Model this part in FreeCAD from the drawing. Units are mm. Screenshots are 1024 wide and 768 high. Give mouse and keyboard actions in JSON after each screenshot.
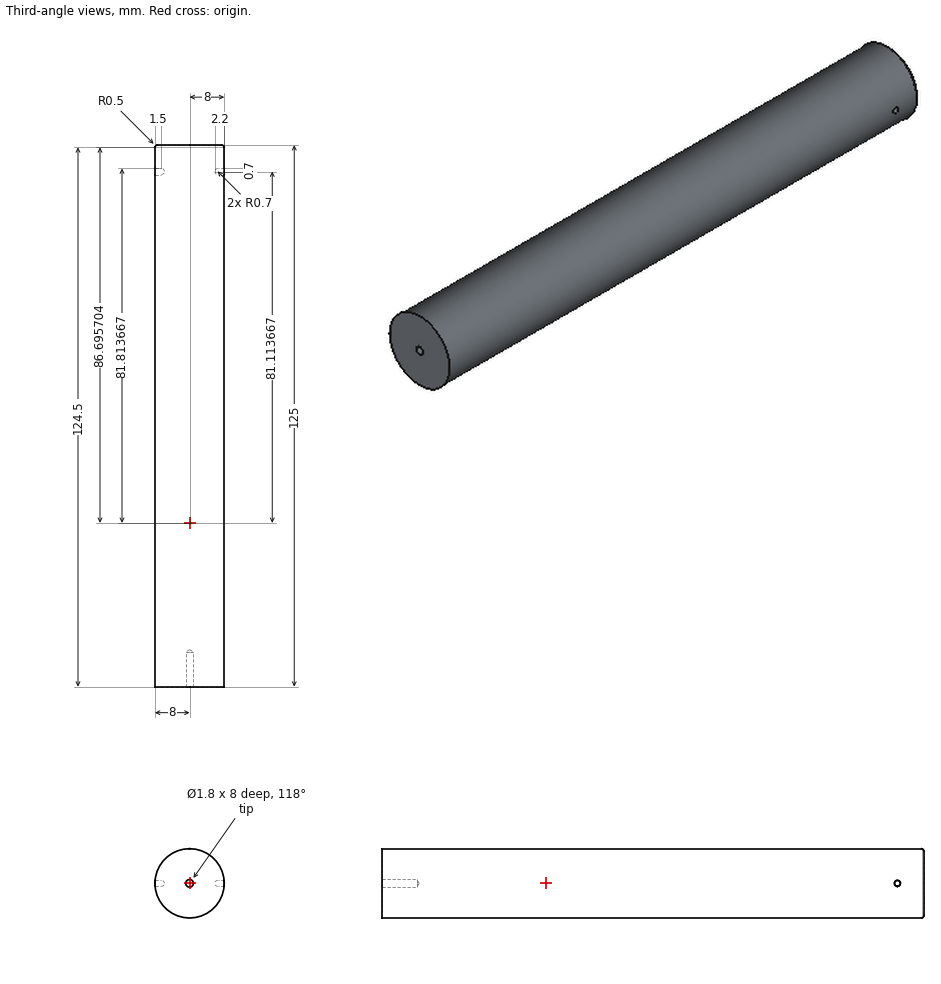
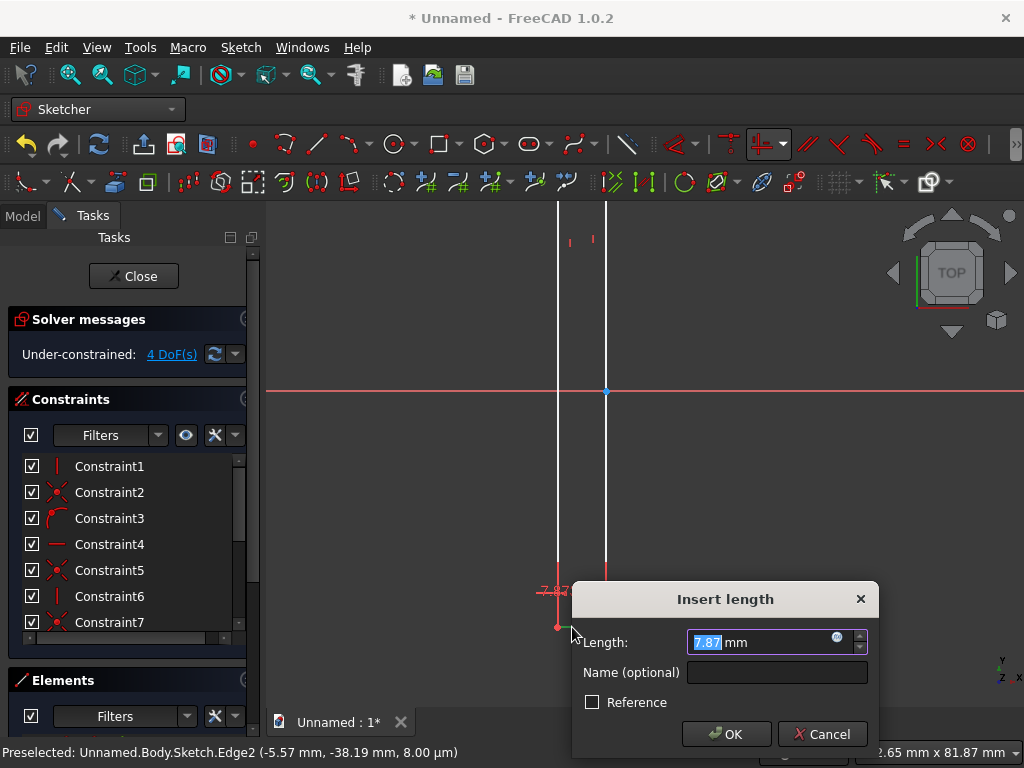
{"action": "type", "text": "8"}
{"action": "key", "text": "Return"}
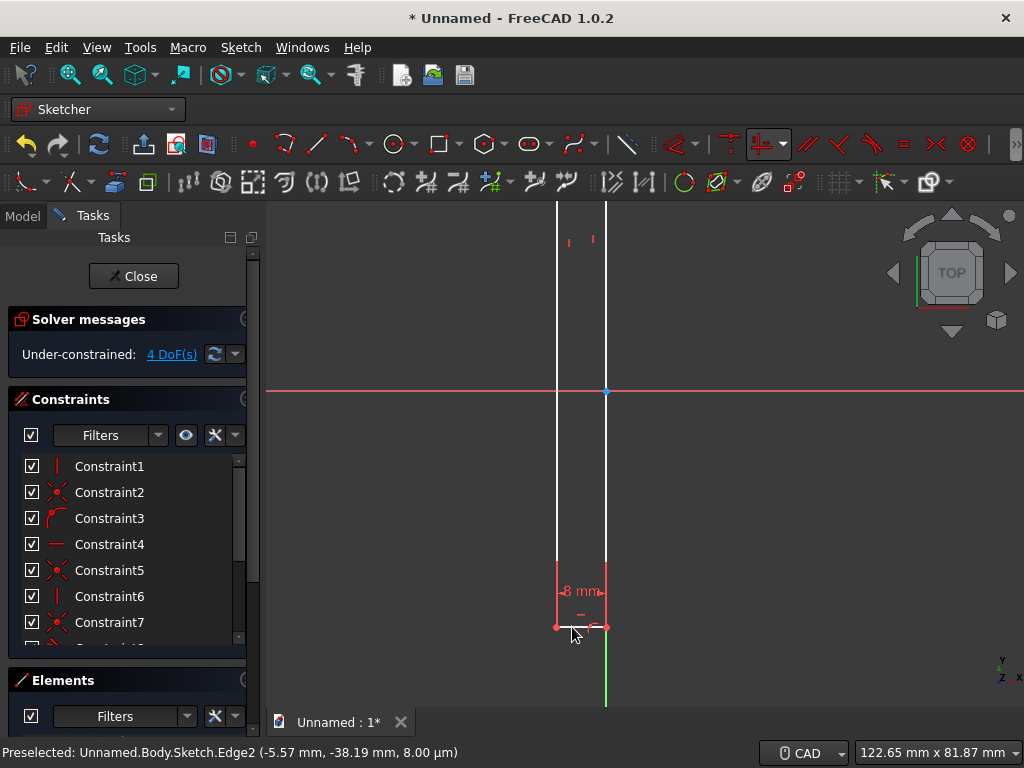
{"action": "left_click", "coordinate": [606, 316]}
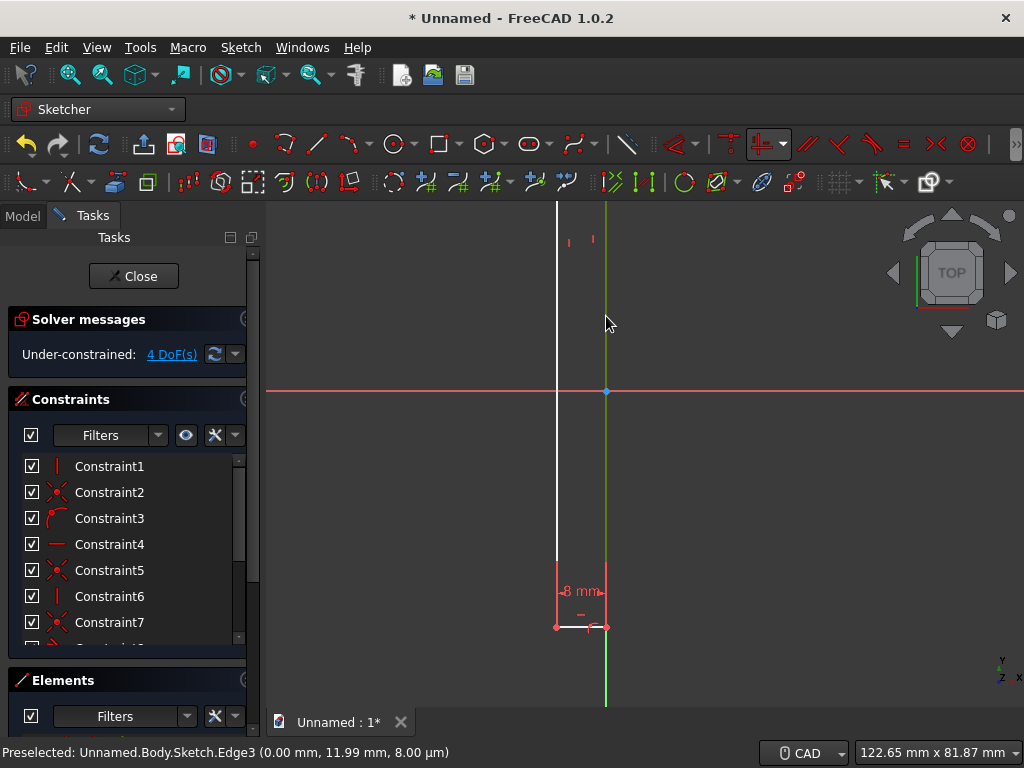
{"action": "key", "text": "i"}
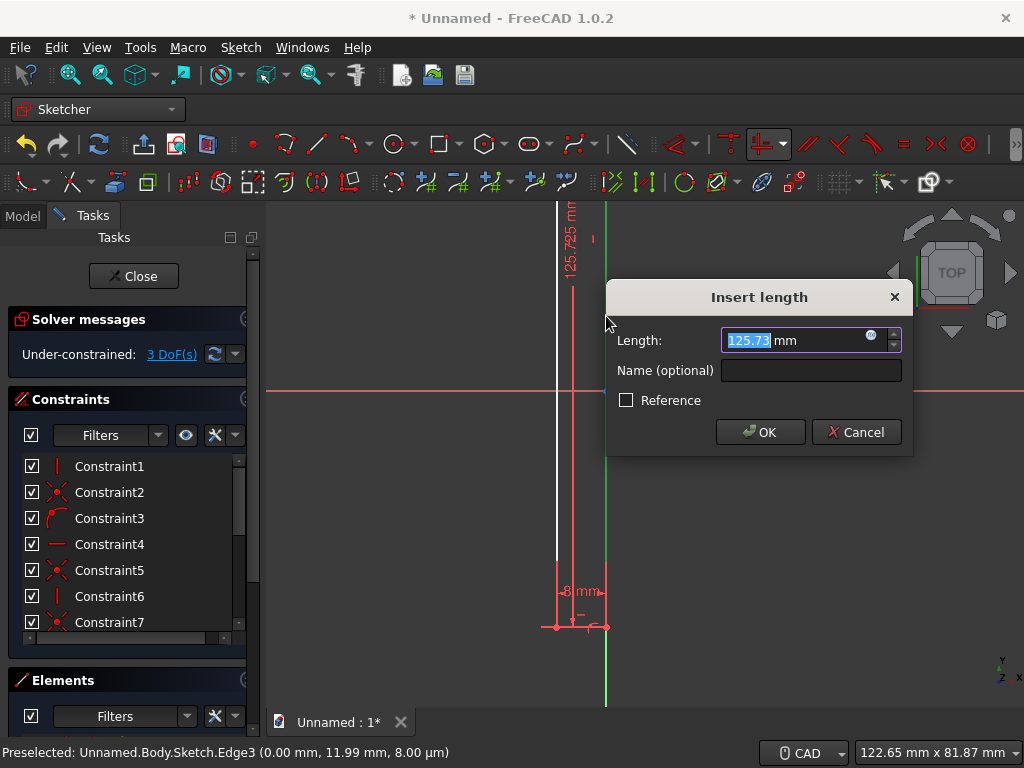
{"action": "type", "text": "125"}
{"action": "key", "text": "Return"}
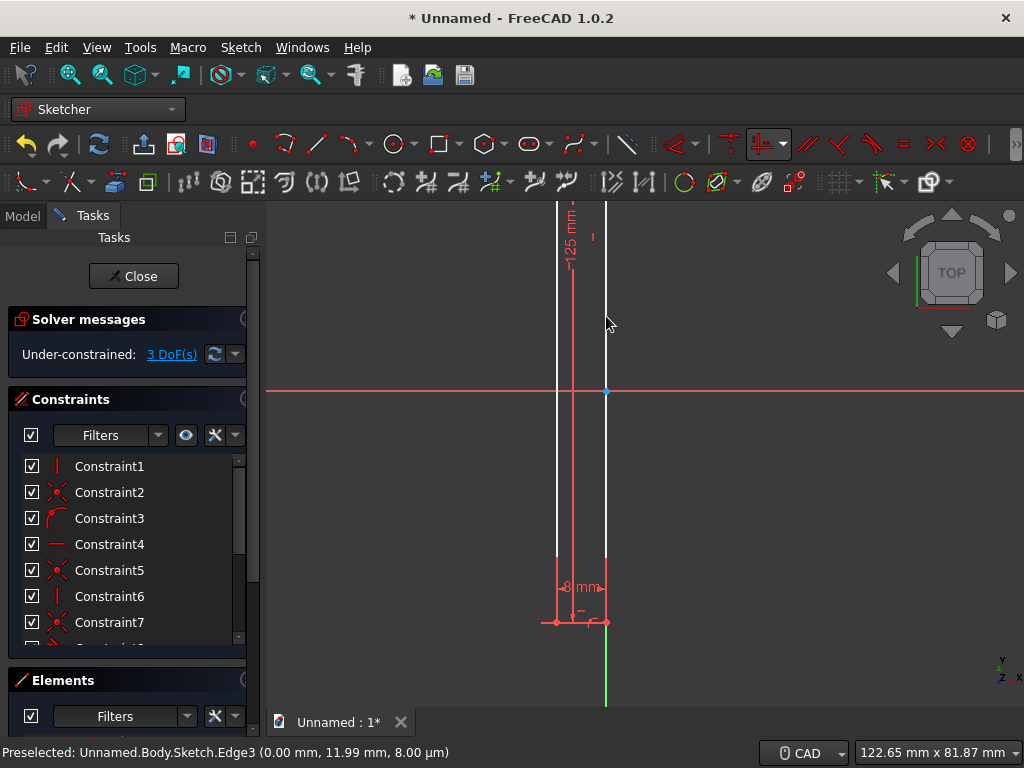
{"action": "left_click", "coordinate": [557, 393]}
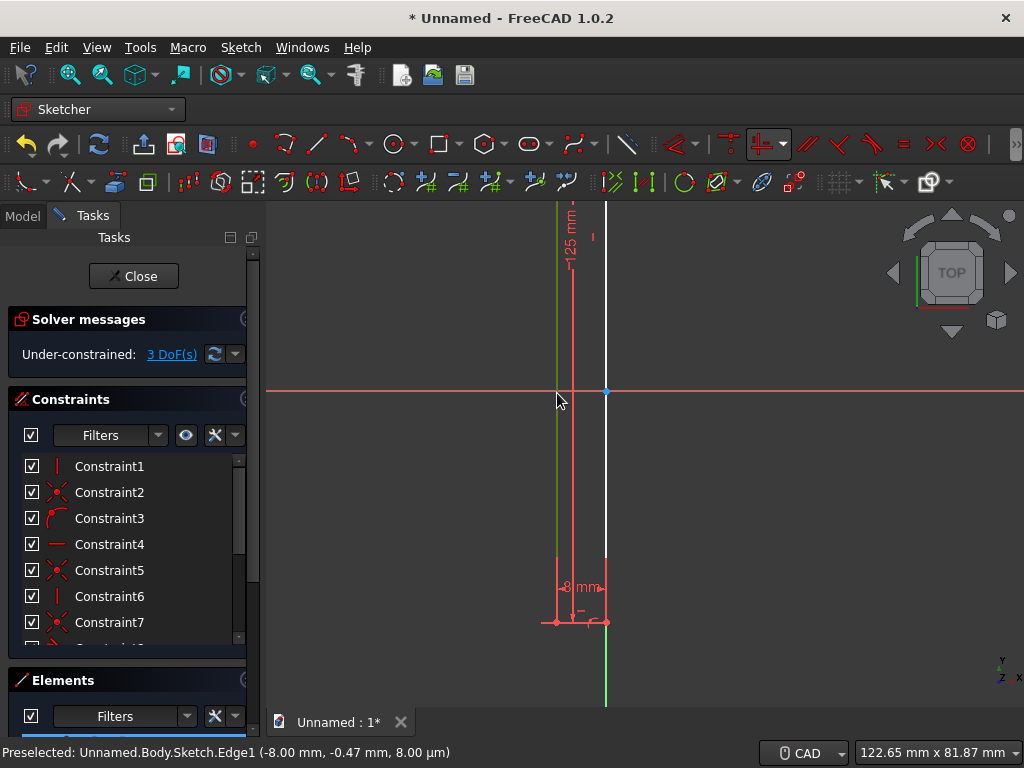
{"action": "key", "text": "i"}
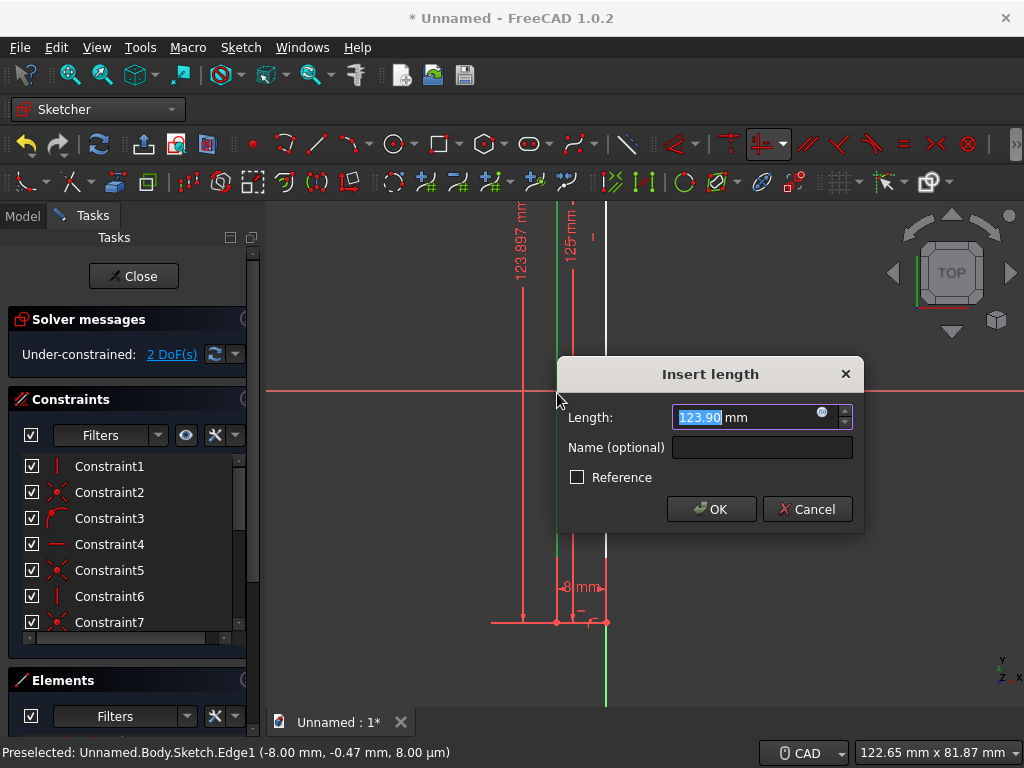
{"action": "type", "text": "124.5"}
{"action": "key", "text": "Return"}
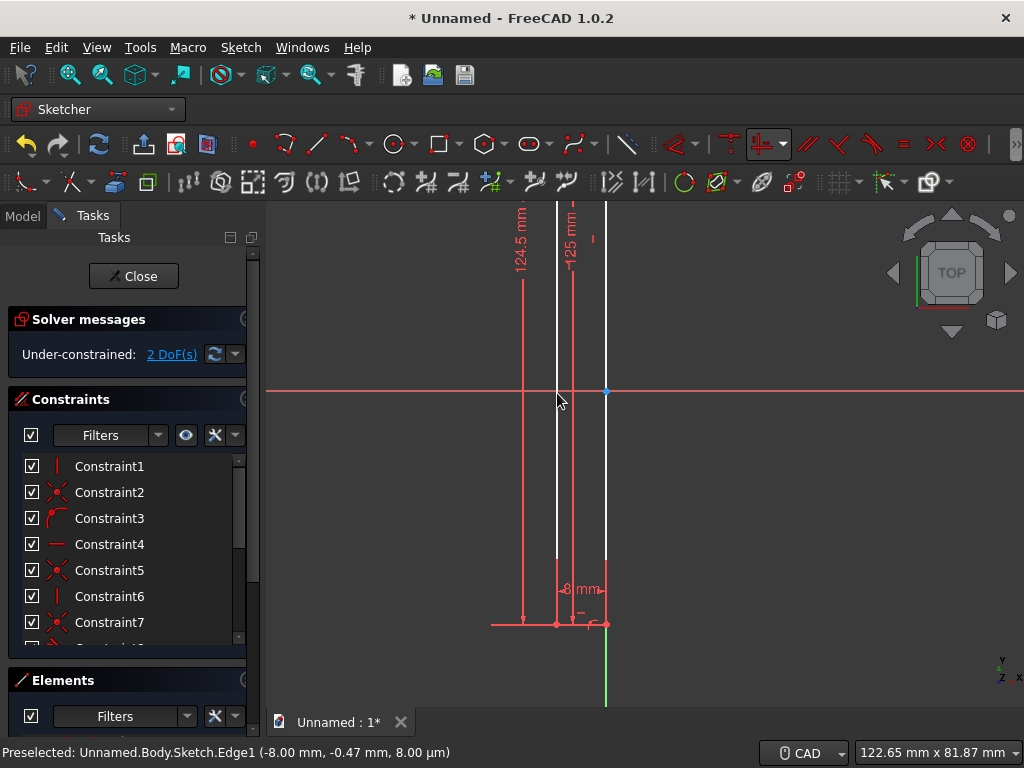
{"action": "scroll", "coordinate": [572, 630], "scroll_direction": "down", "scroll_amount": 4}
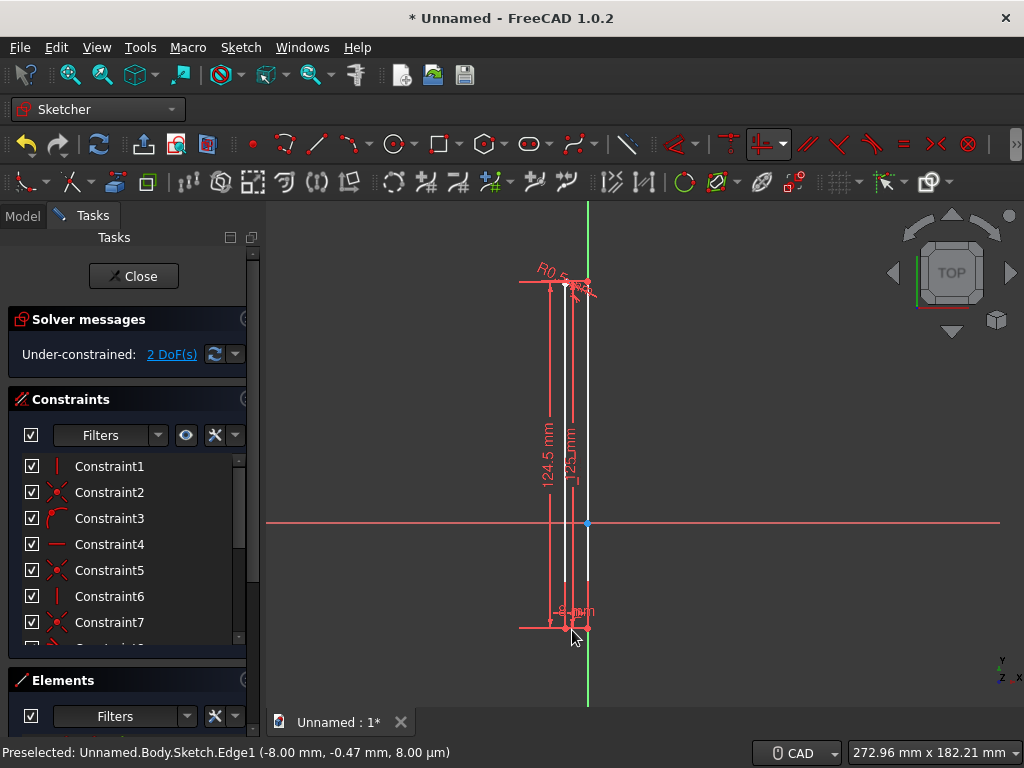
{"action": "scroll", "coordinate": [565, 282], "scroll_direction": "up", "scroll_amount": 11}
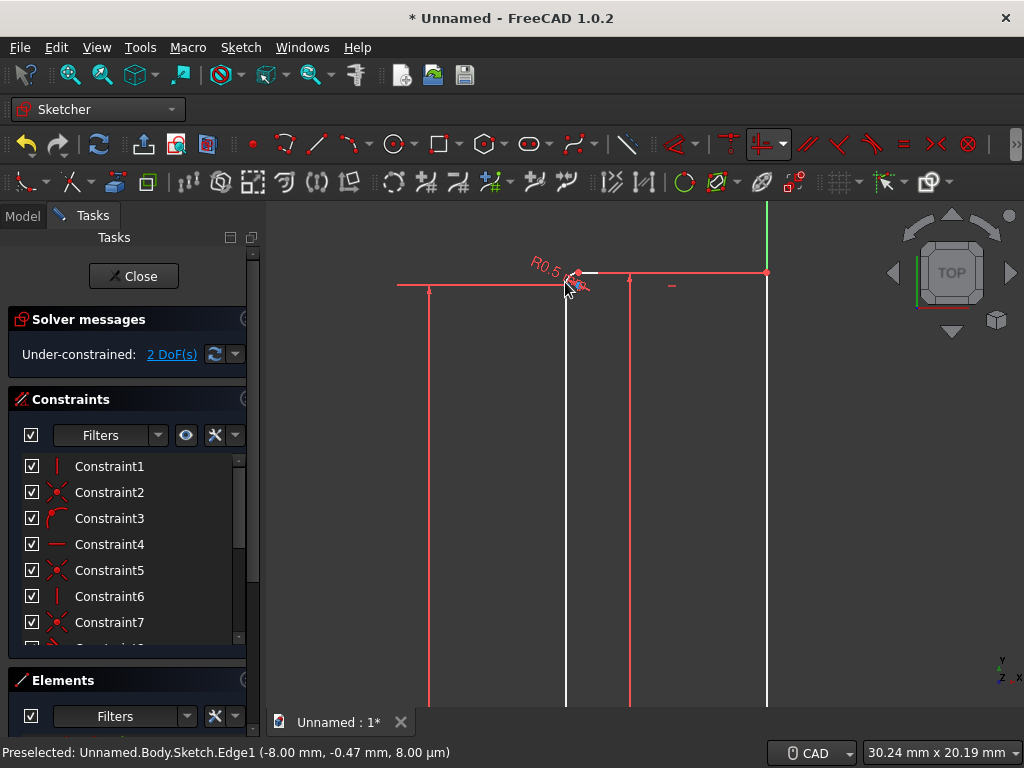
{"action": "left_click", "coordinate": [566, 285]}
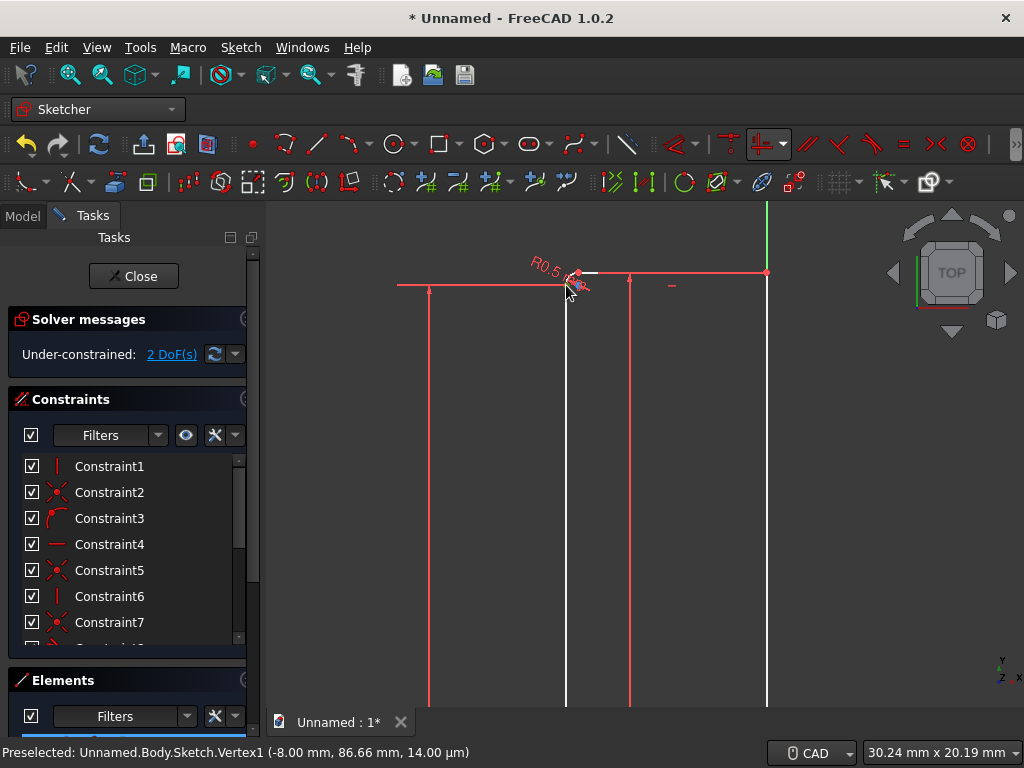
{"action": "key", "text": "i"}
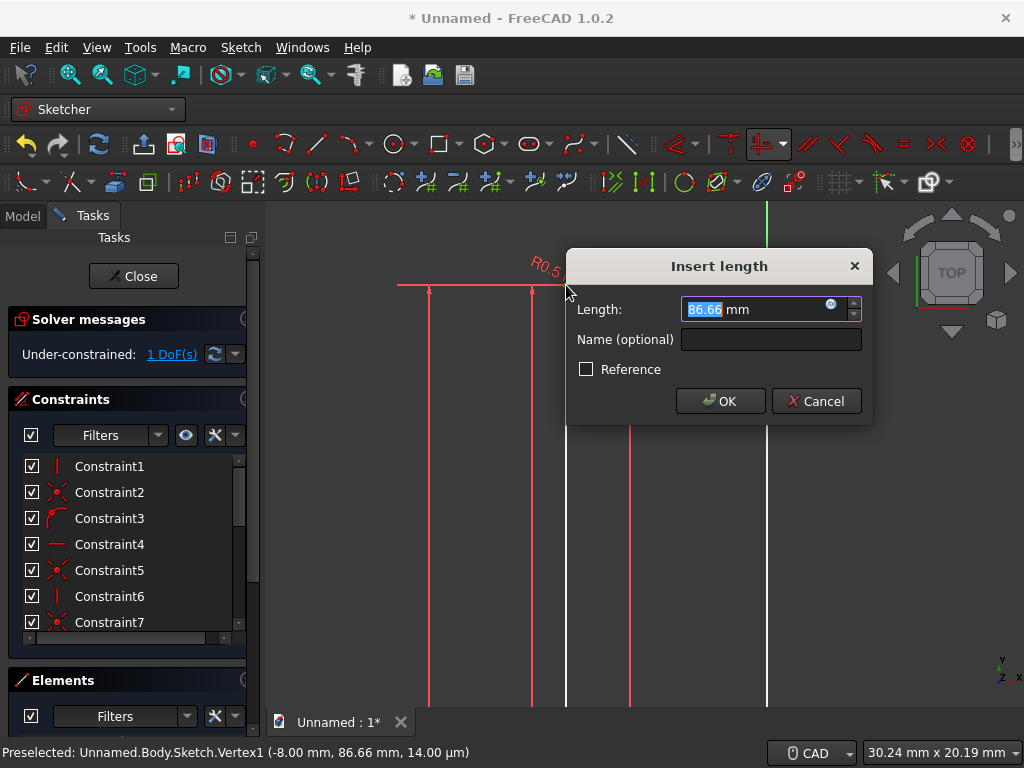
{"action": "type", "text": "86.695704"}
{"action": "key", "text": "Return"}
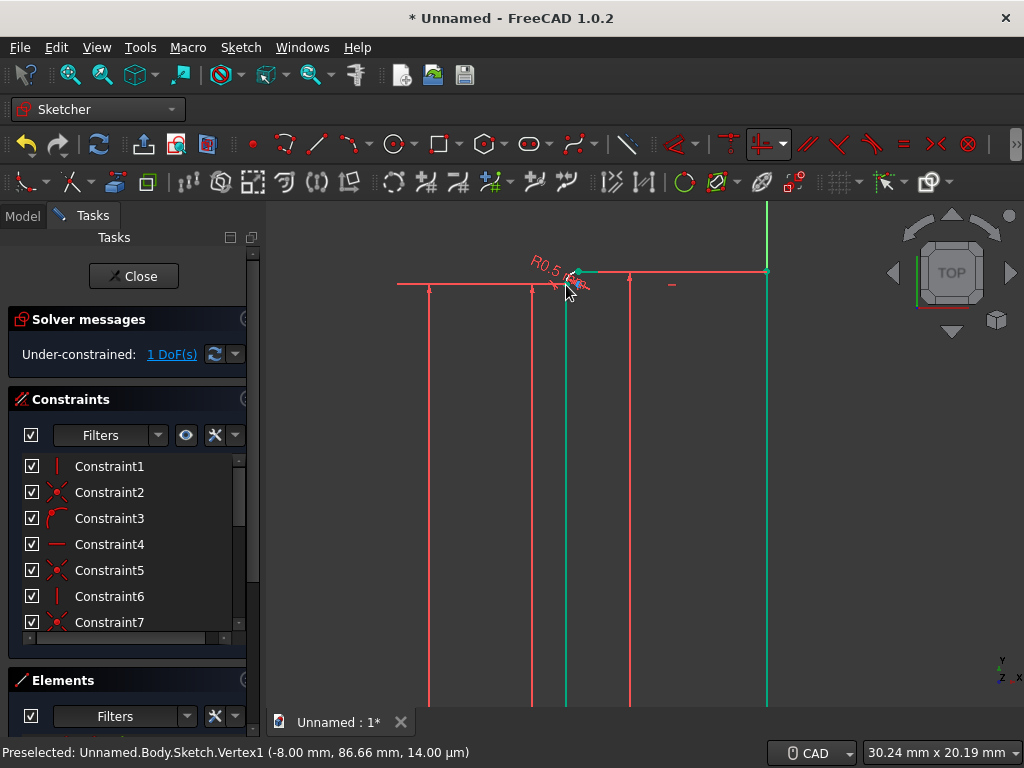
{"action": "left_click", "coordinate": [569, 292]}